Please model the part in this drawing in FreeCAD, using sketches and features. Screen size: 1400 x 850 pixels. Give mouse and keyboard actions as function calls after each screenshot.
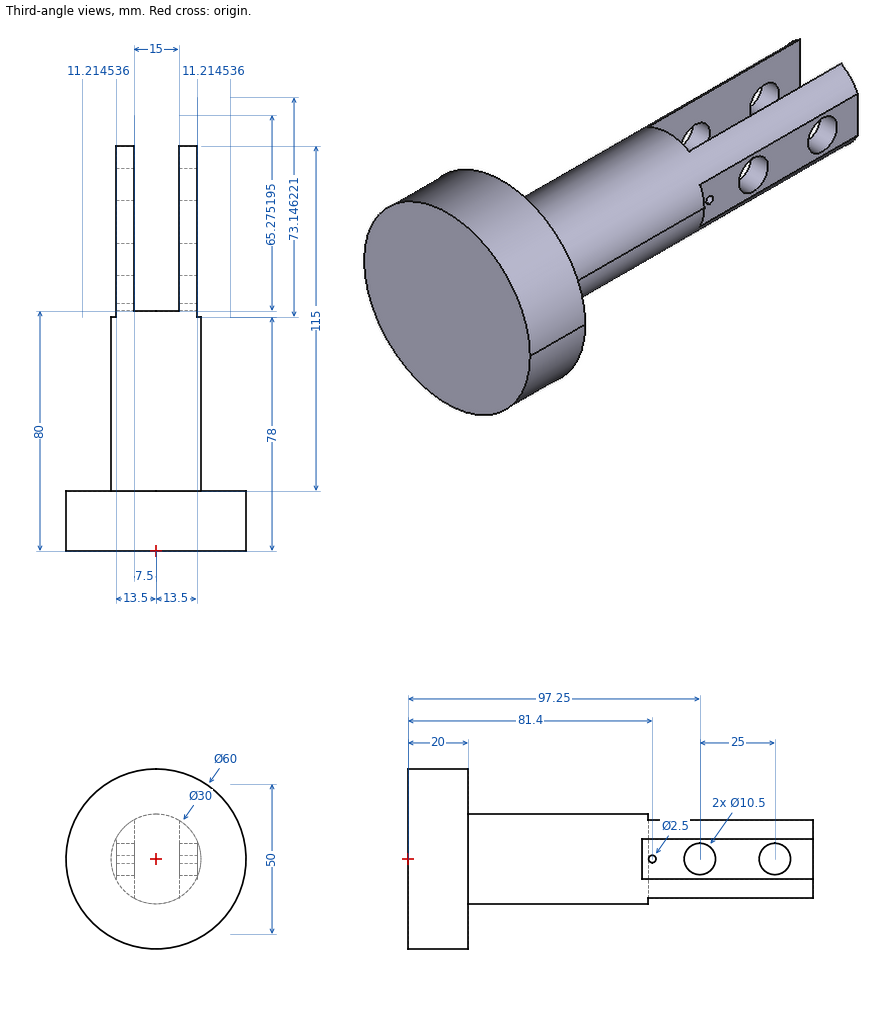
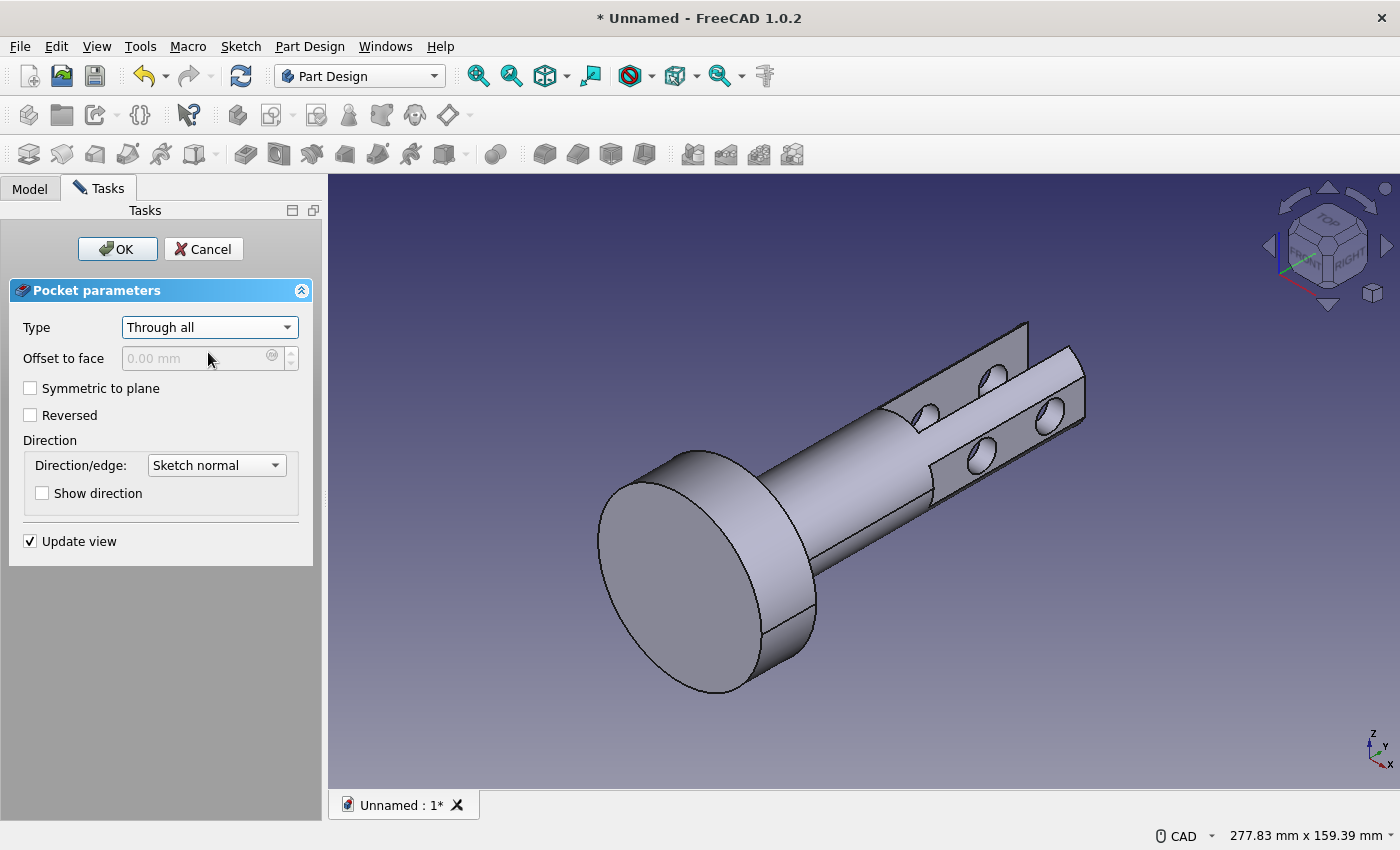
click(118, 249)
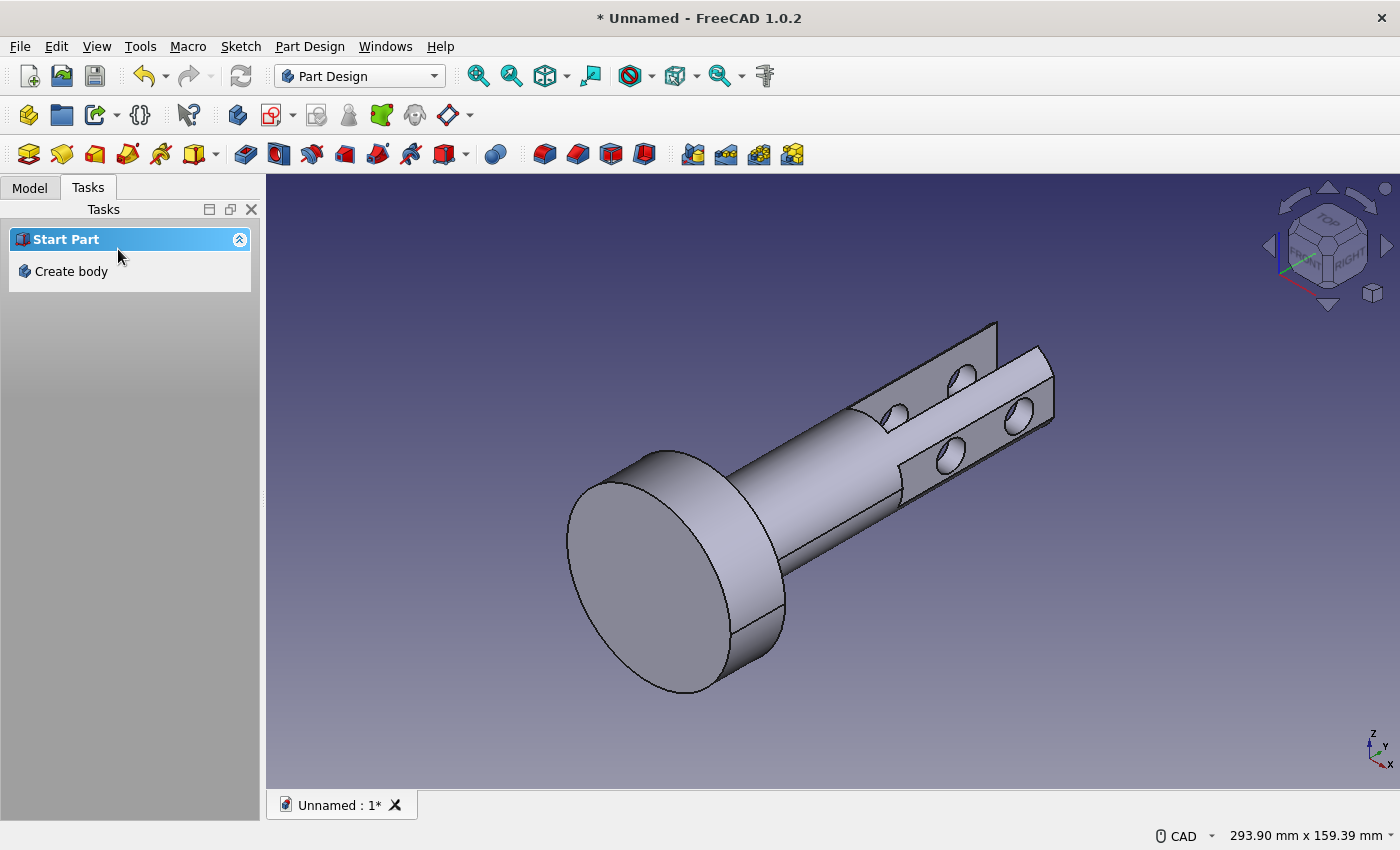
key(6)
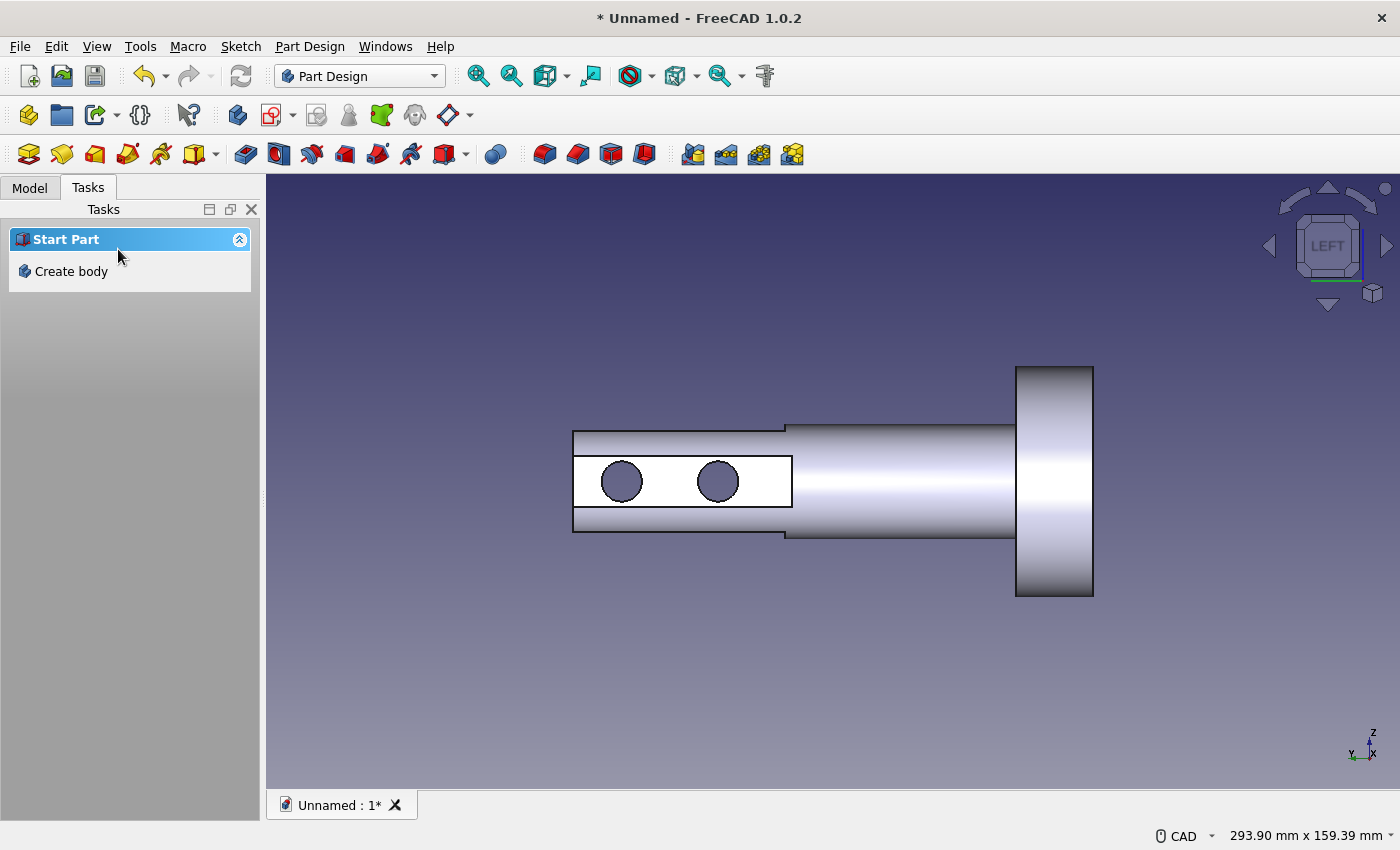
click(683, 473)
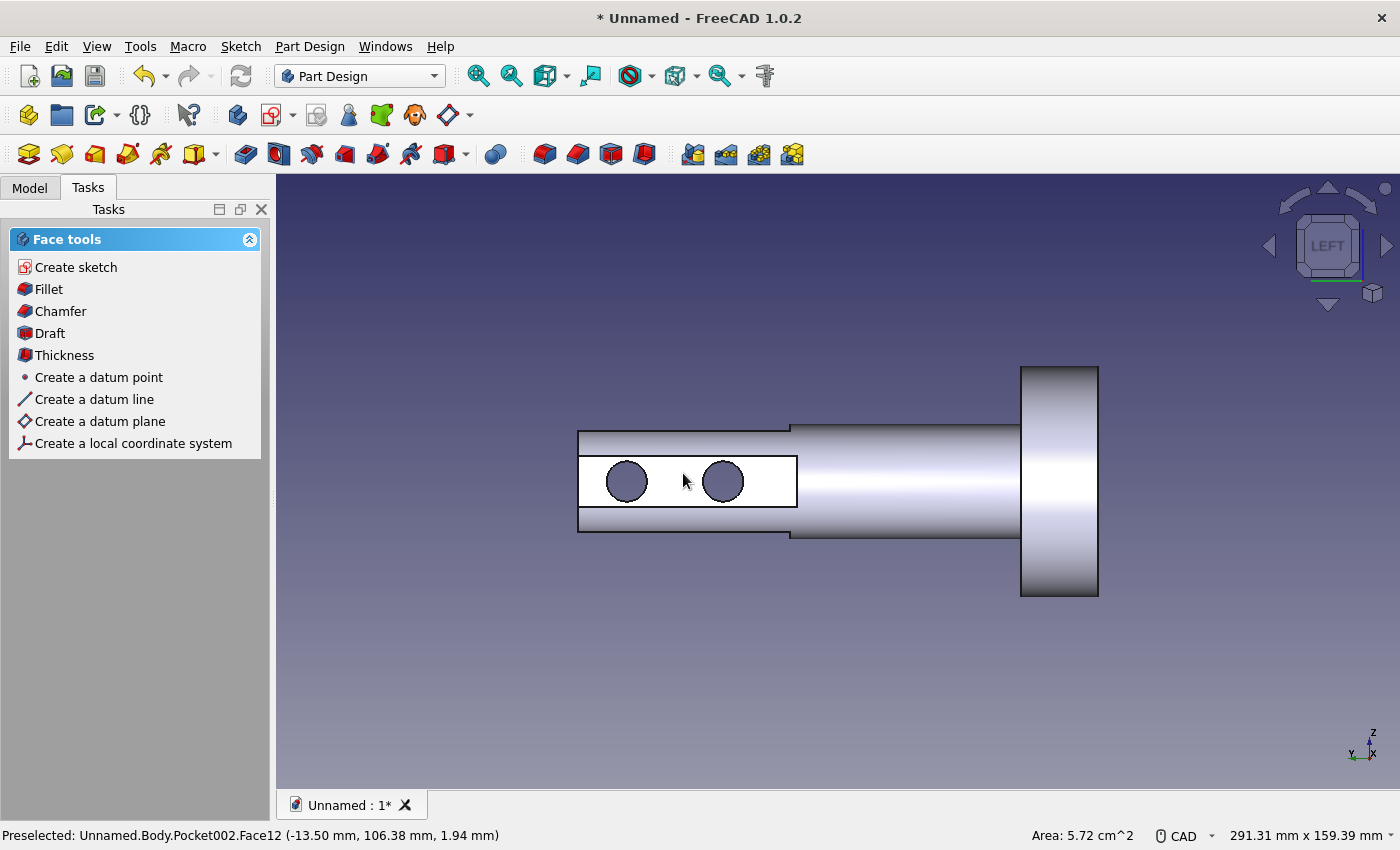
click(270, 116)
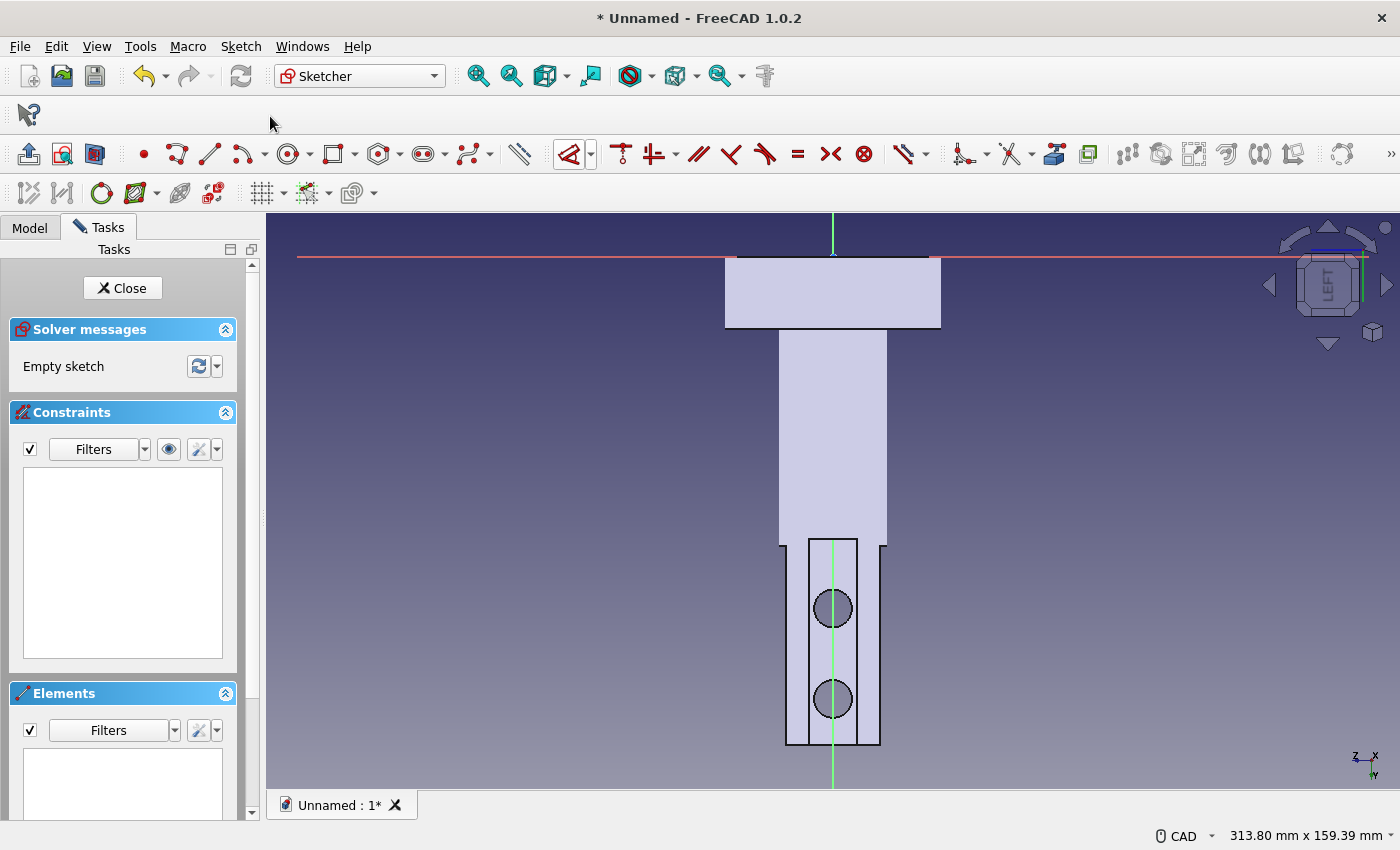
click(95, 154)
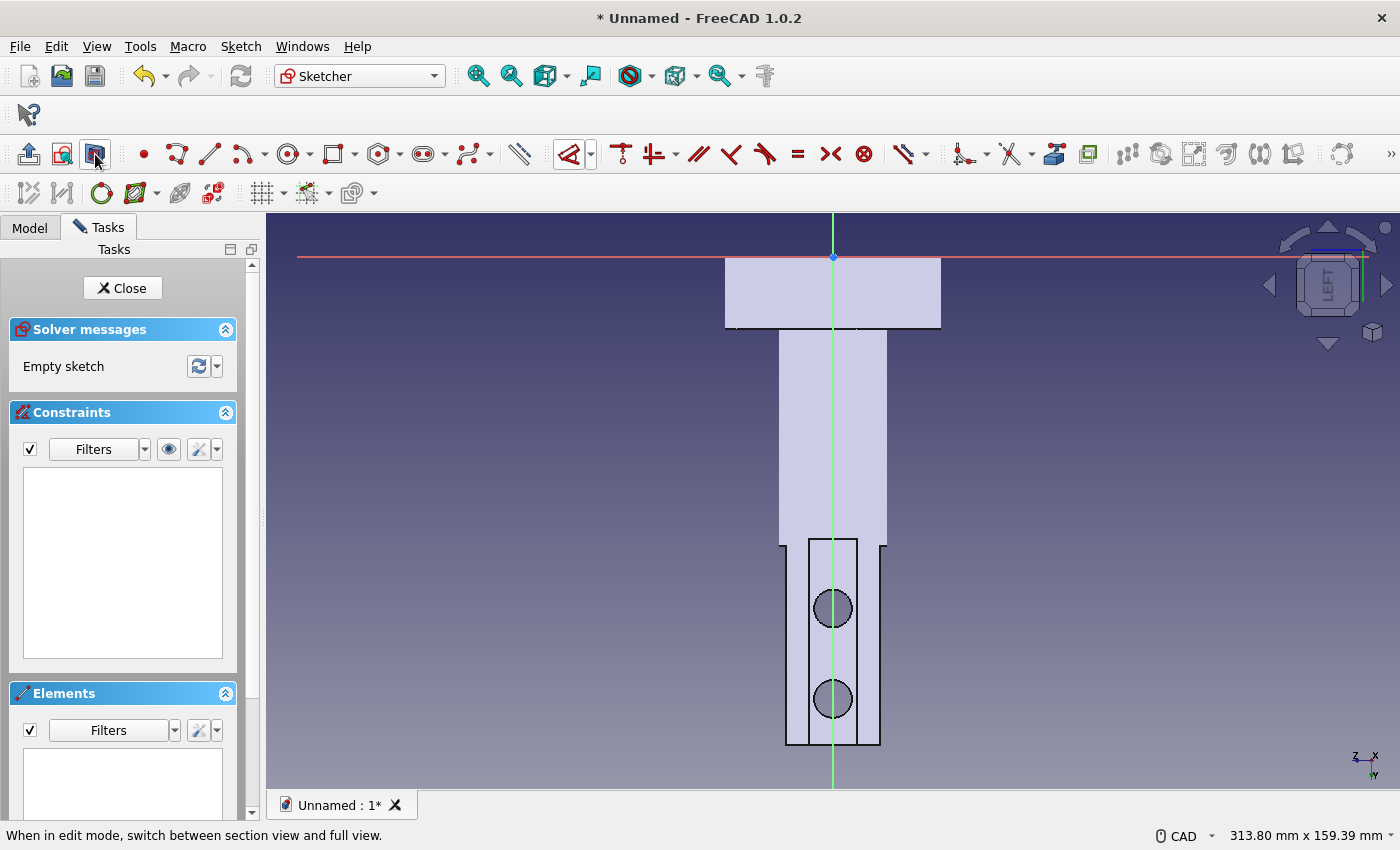
scroll(837, 554, up, 15)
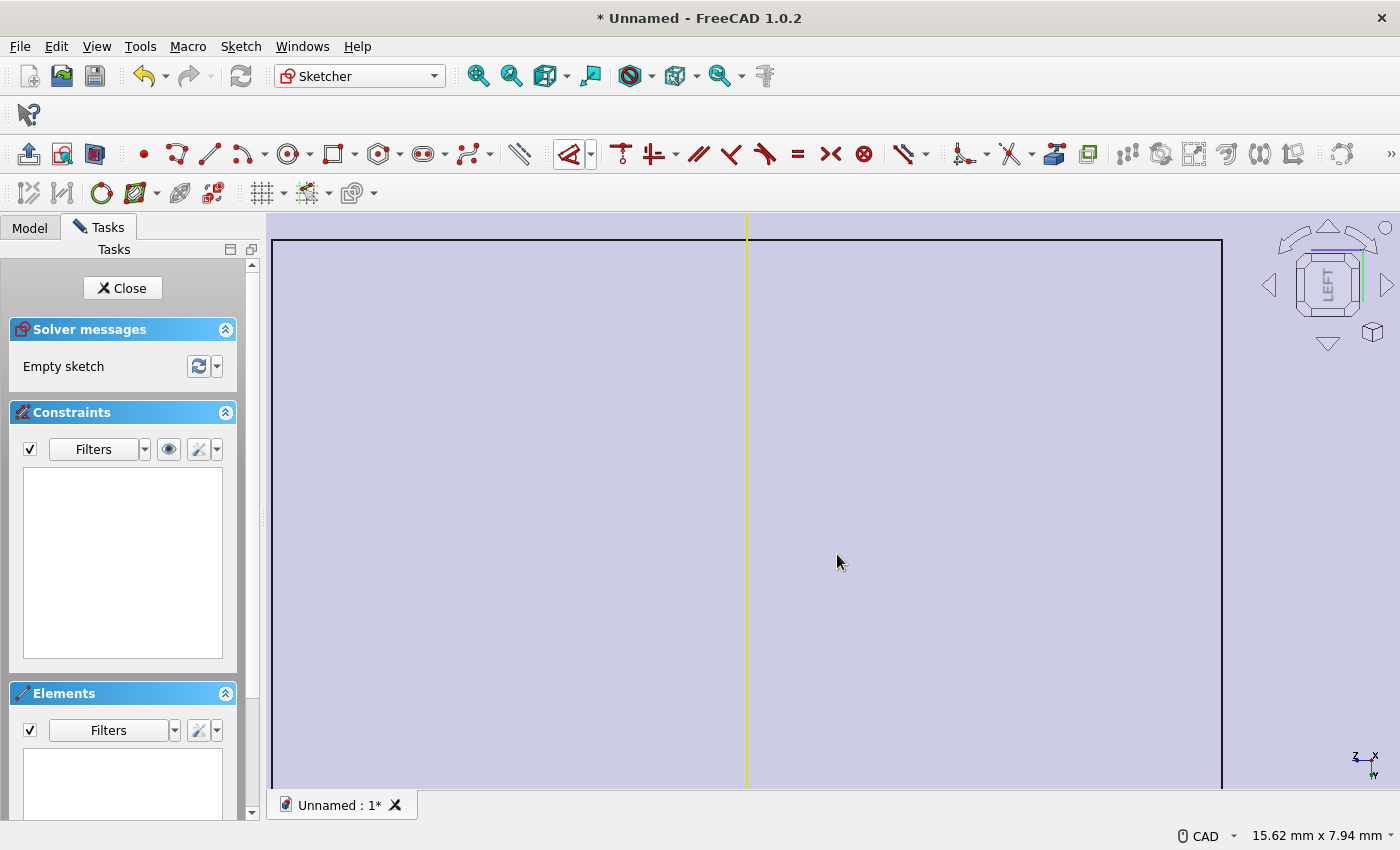
scroll(733, 476, up, 4)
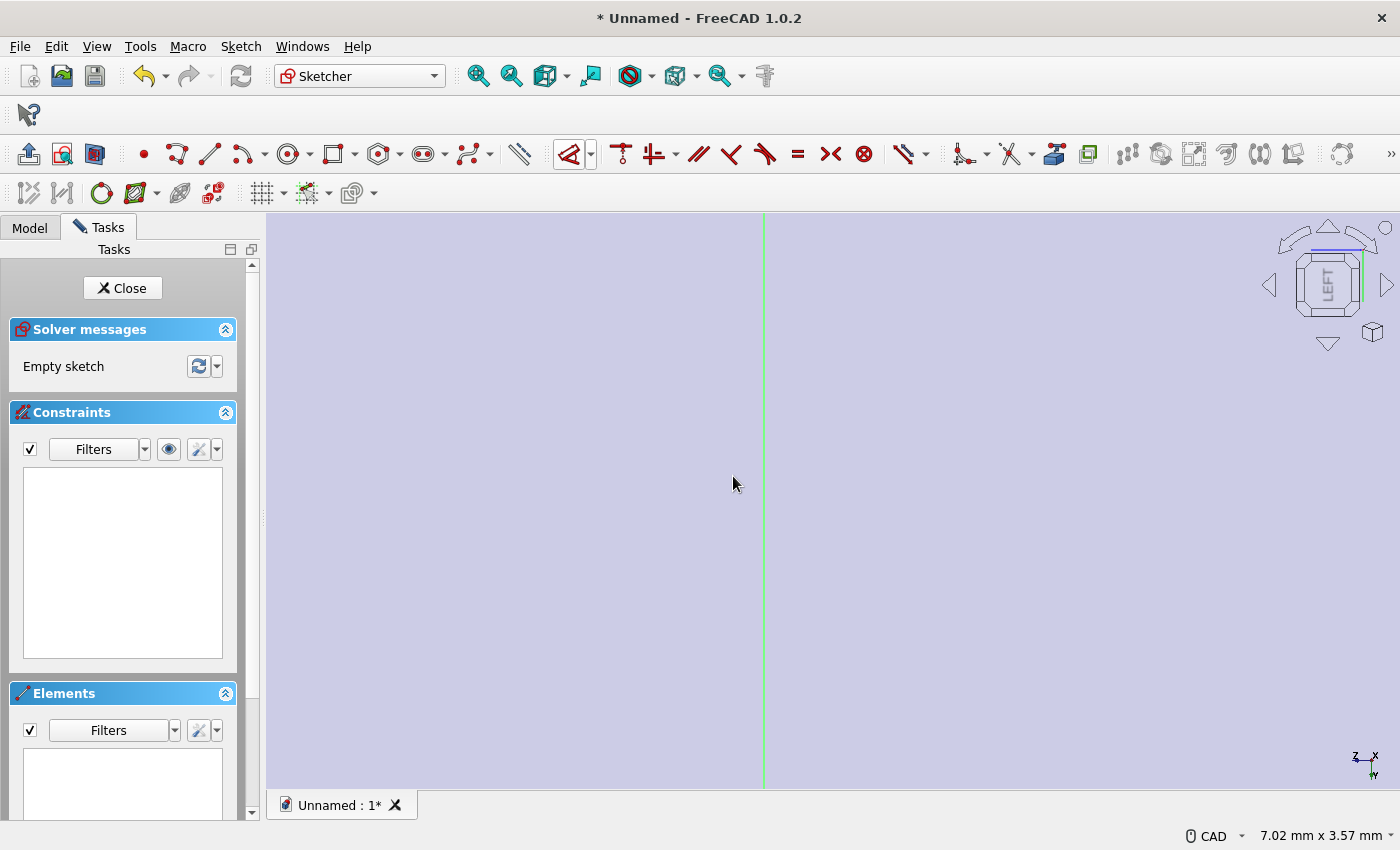
click(288, 154)